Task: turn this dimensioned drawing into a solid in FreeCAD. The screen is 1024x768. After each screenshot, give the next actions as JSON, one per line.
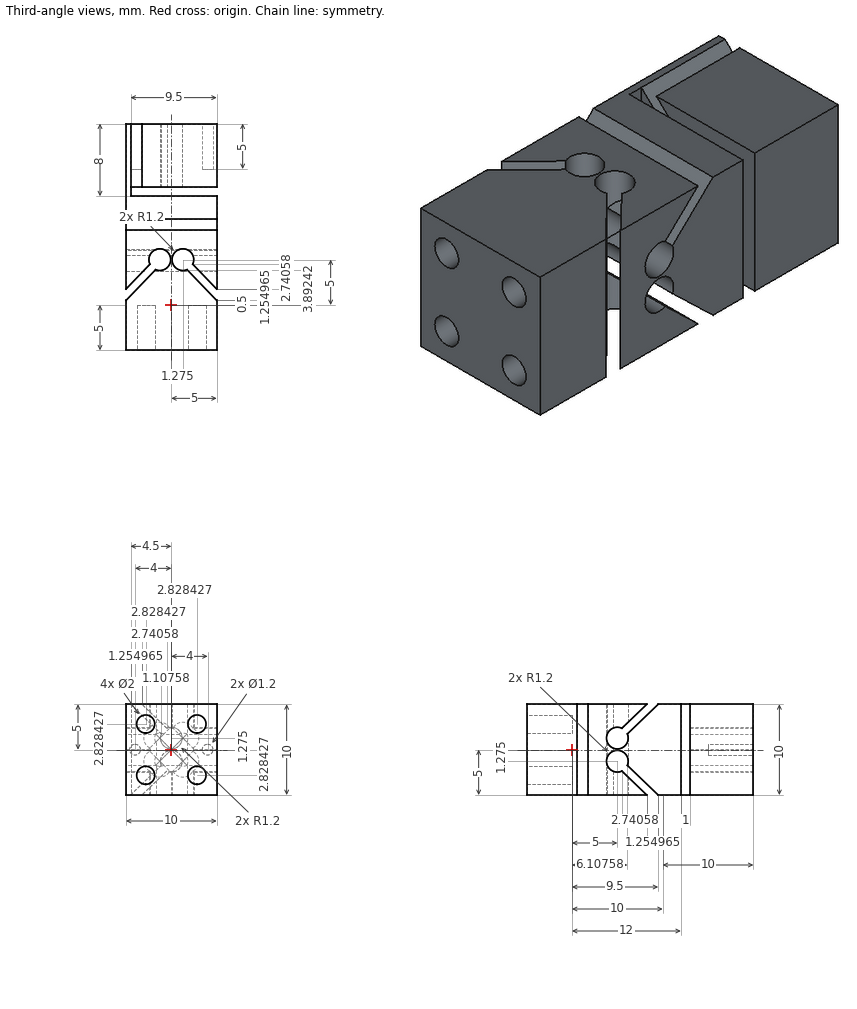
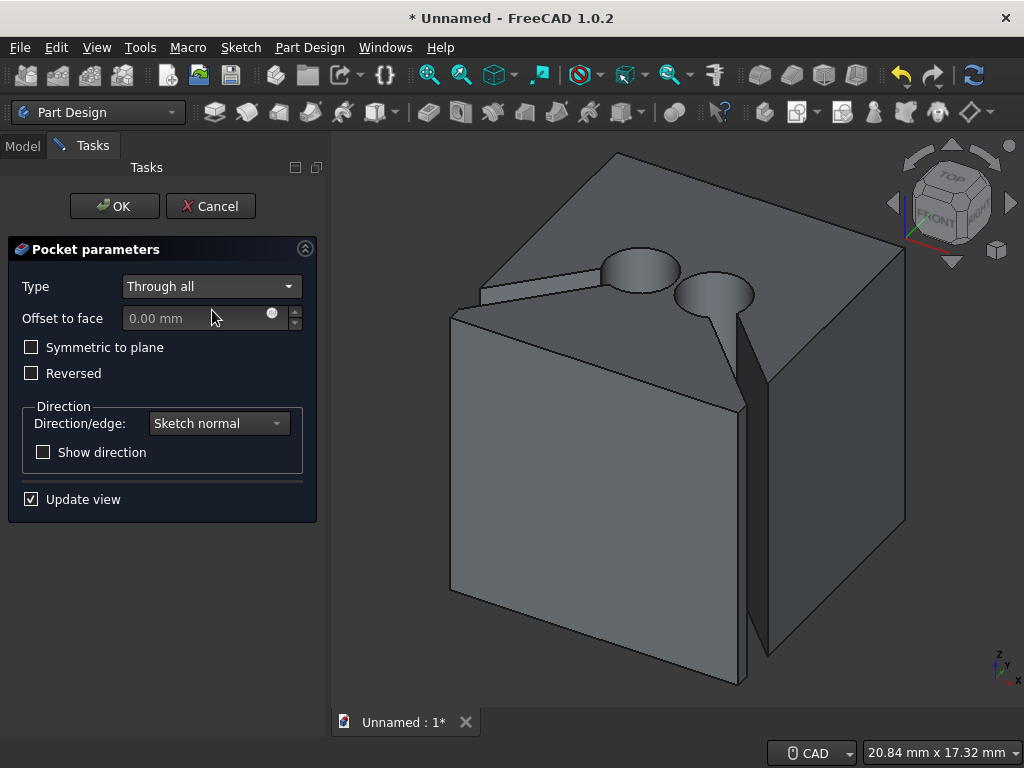
{"action": "left_click", "coordinate": [115, 206]}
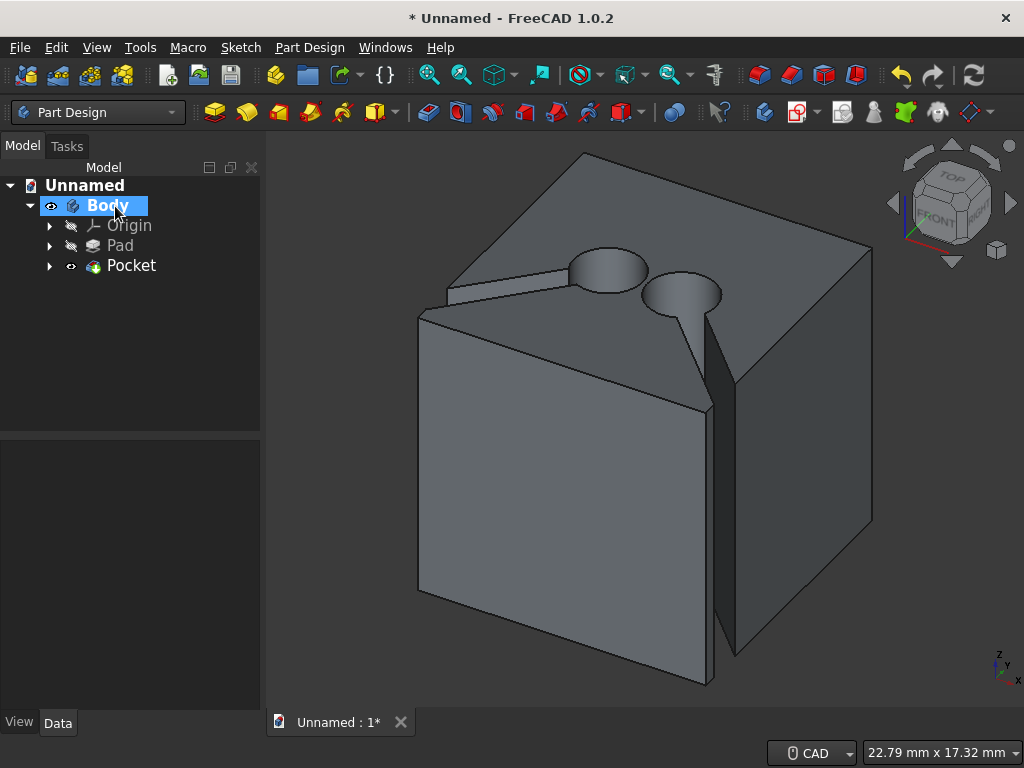
{"action": "left_click", "coordinate": [804, 451]}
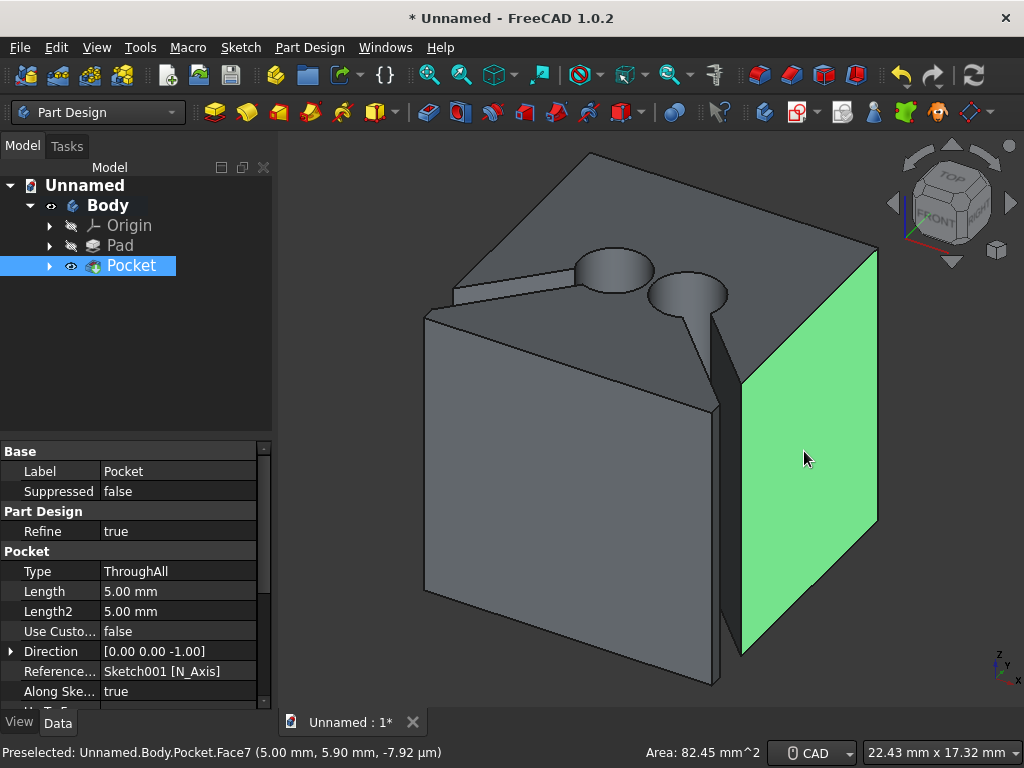
{"action": "left_click", "coordinate": [798, 112]}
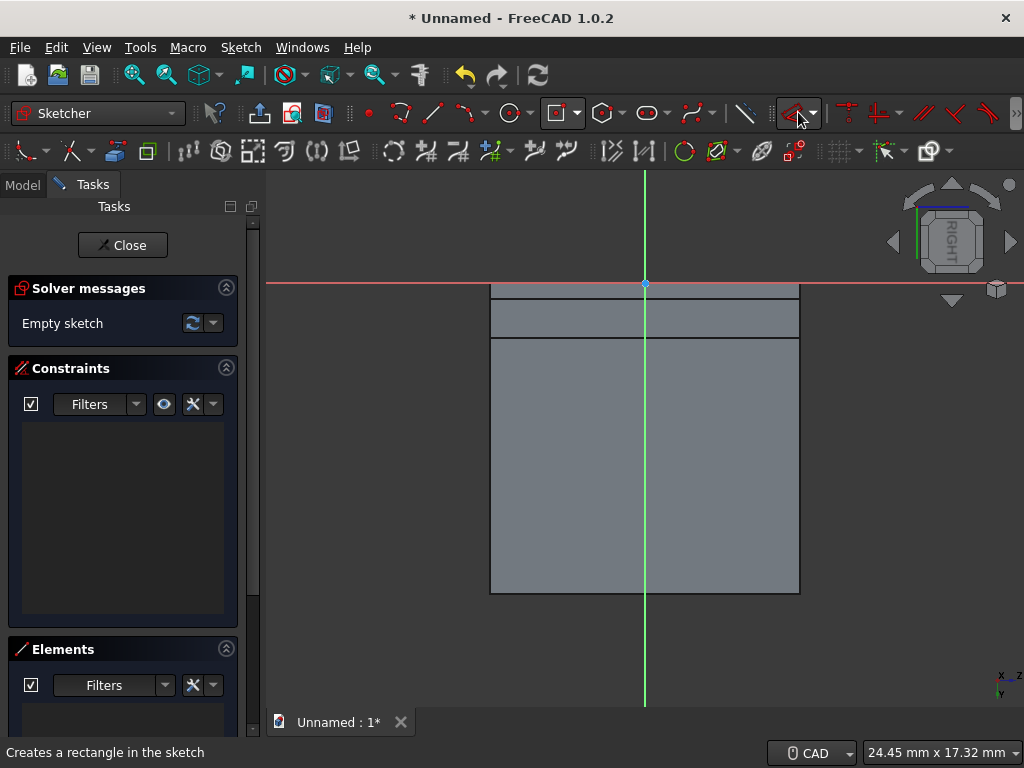
{"action": "left_click", "coordinate": [402, 114]}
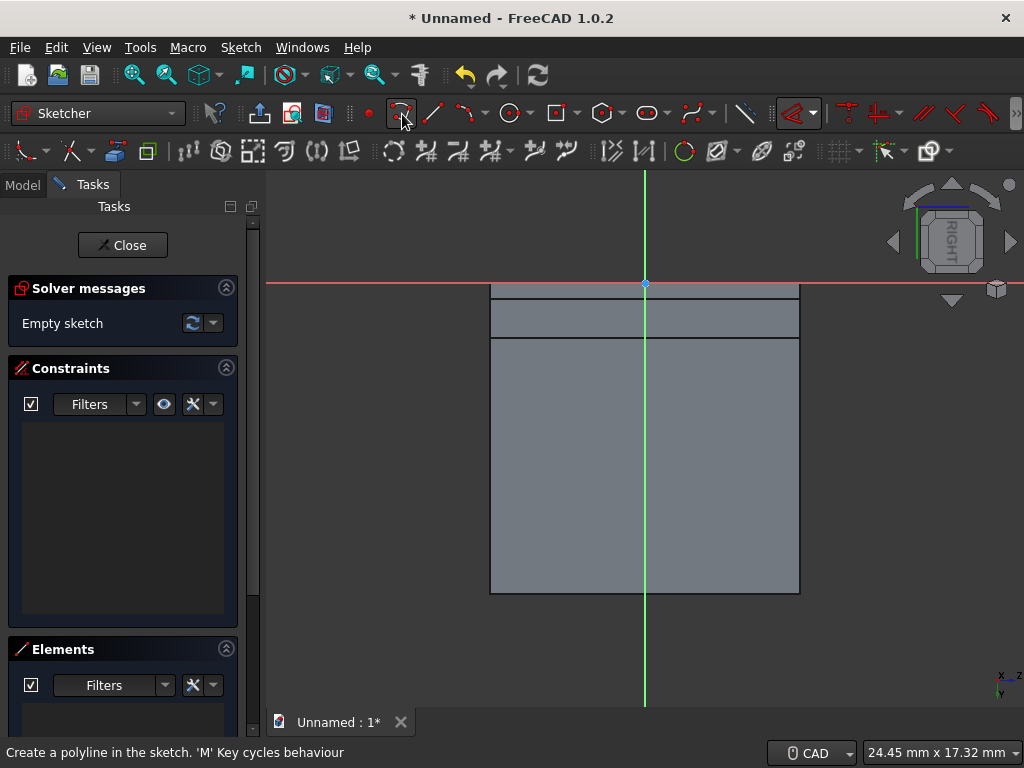
{"action": "left_click", "coordinate": [572, 454]}
{"action": "left_click", "coordinate": [490, 539]}
{"action": "left_click", "coordinate": [490, 578]}
{"action": "left_click", "coordinate": [591, 473]}
{"action": "right_click", "coordinate": [591, 473]}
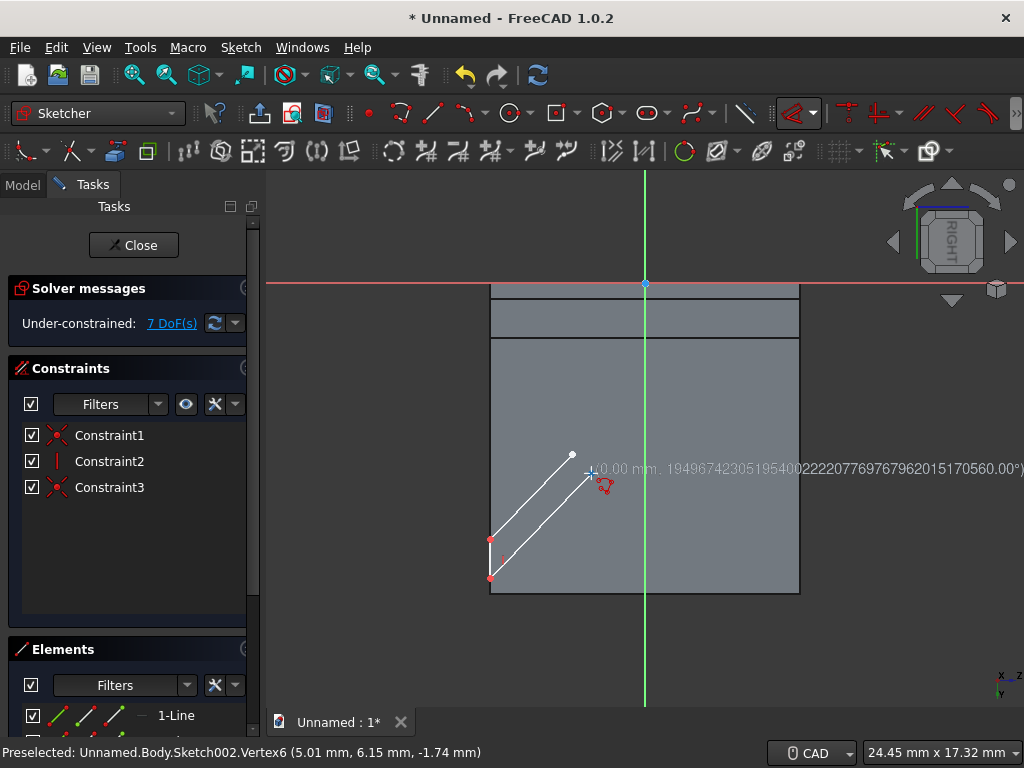
{"action": "left_click", "coordinate": [466, 114]}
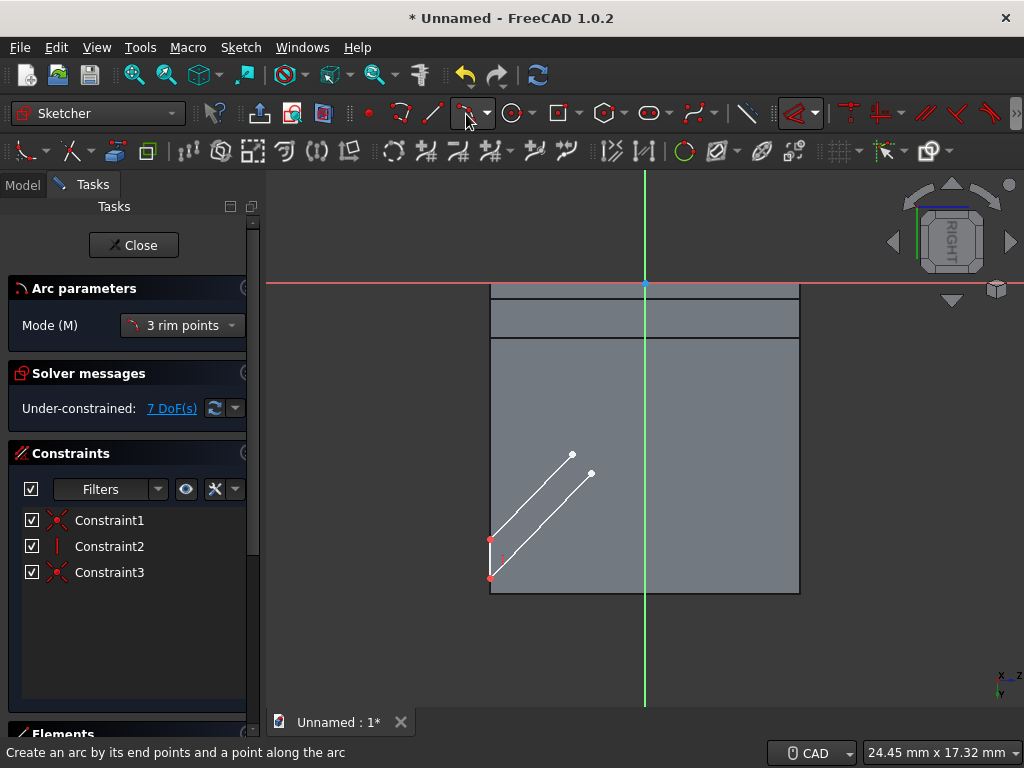
{"action": "left_click", "coordinate": [591, 474]}
{"action": "left_click", "coordinate": [572, 455]}
{"action": "left_click", "coordinate": [613, 402]}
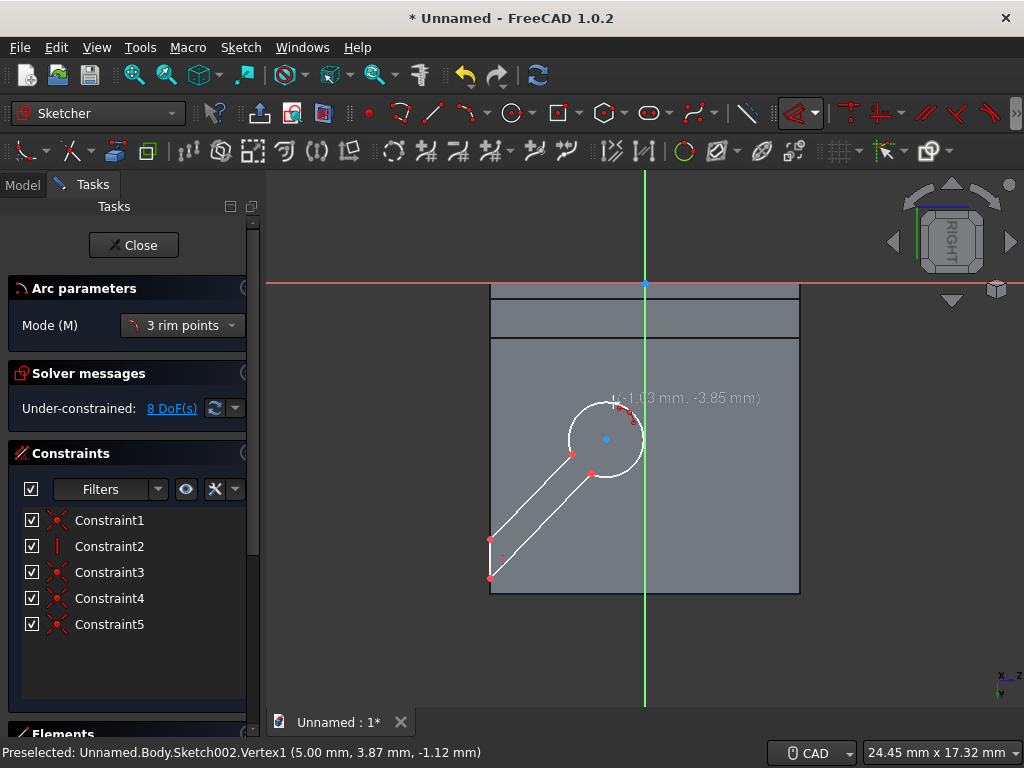
{"action": "left_click", "coordinate": [402, 114]}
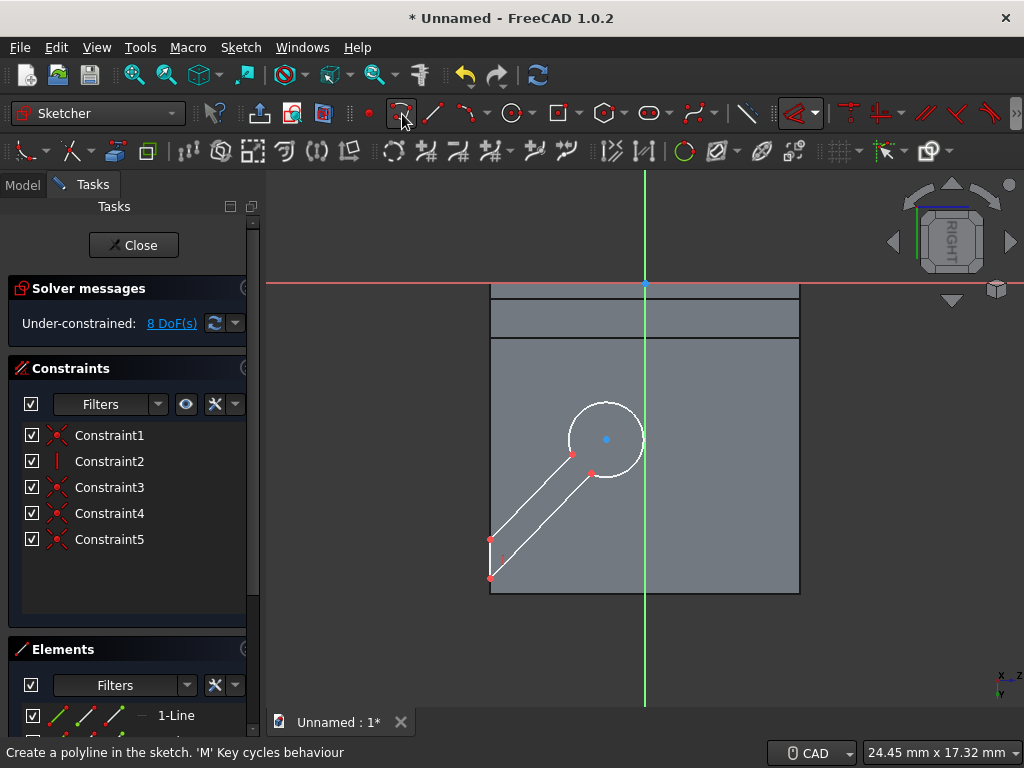
{"action": "left_click", "coordinate": [699, 473]}
{"action": "left_click", "coordinate": [800, 578]}
{"action": "left_click", "coordinate": [800, 539]}
{"action": "left_click", "coordinate": [718, 454]}
{"action": "right_click", "coordinate": [718, 454]}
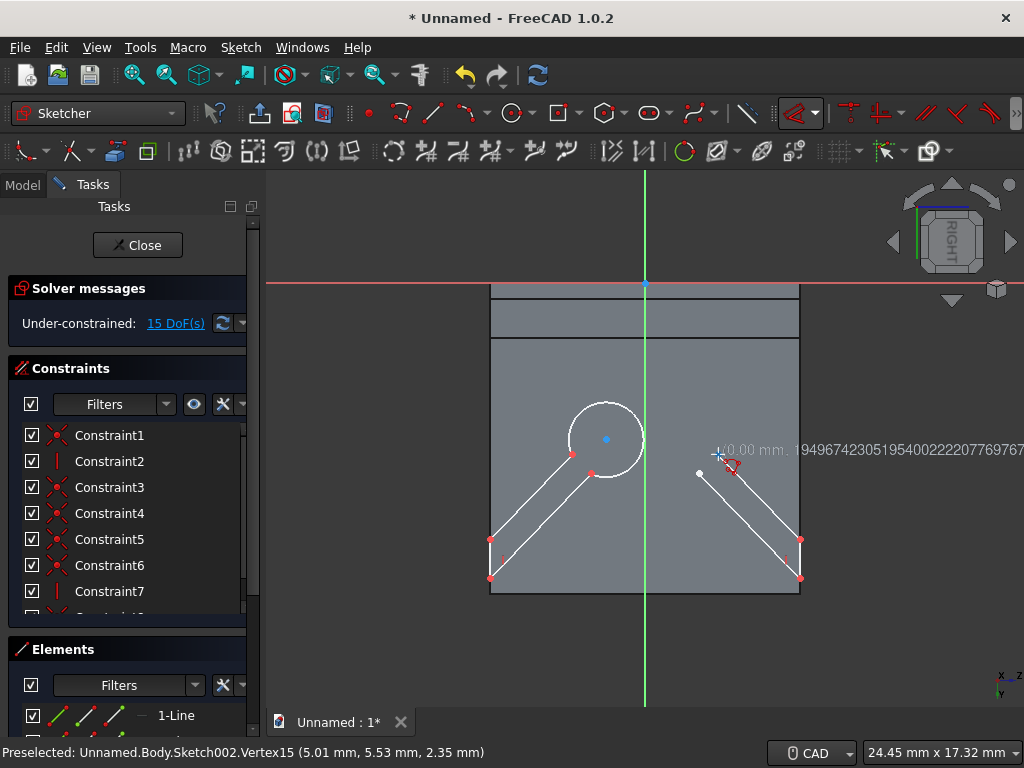
{"action": "left_click", "coordinate": [466, 114]}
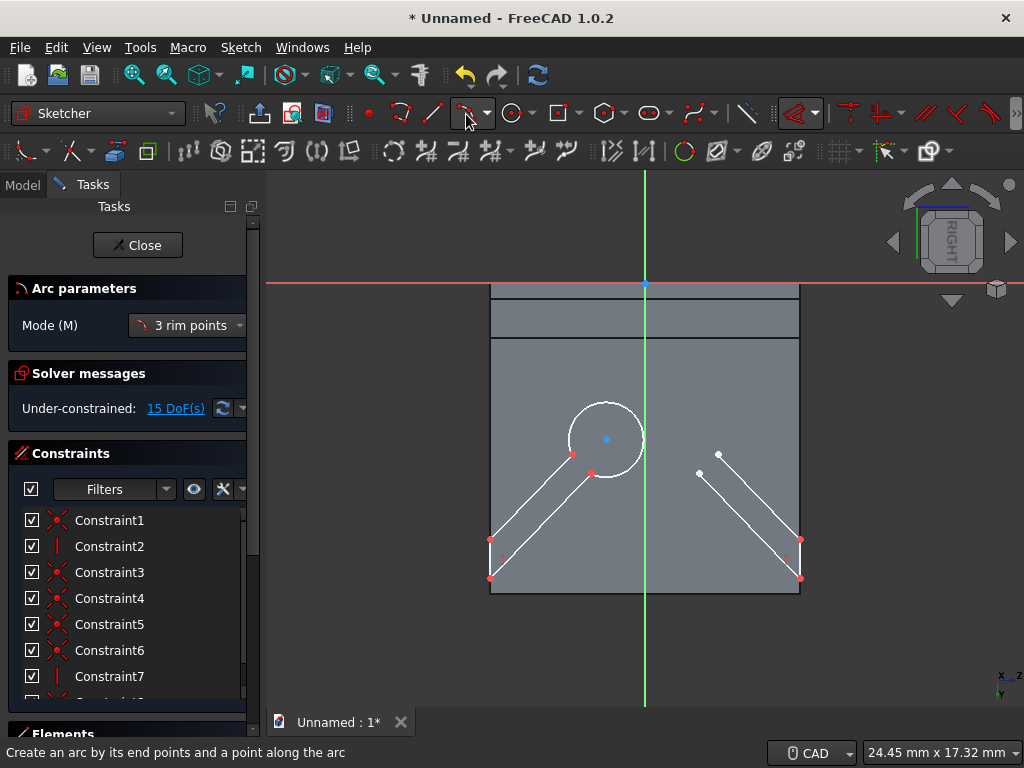
{"action": "left_click", "coordinate": [718, 455]}
{"action": "left_click", "coordinate": [699, 474]}
{"action": "left_click", "coordinate": [677, 402]}
{"action": "key", "text": "Escape"}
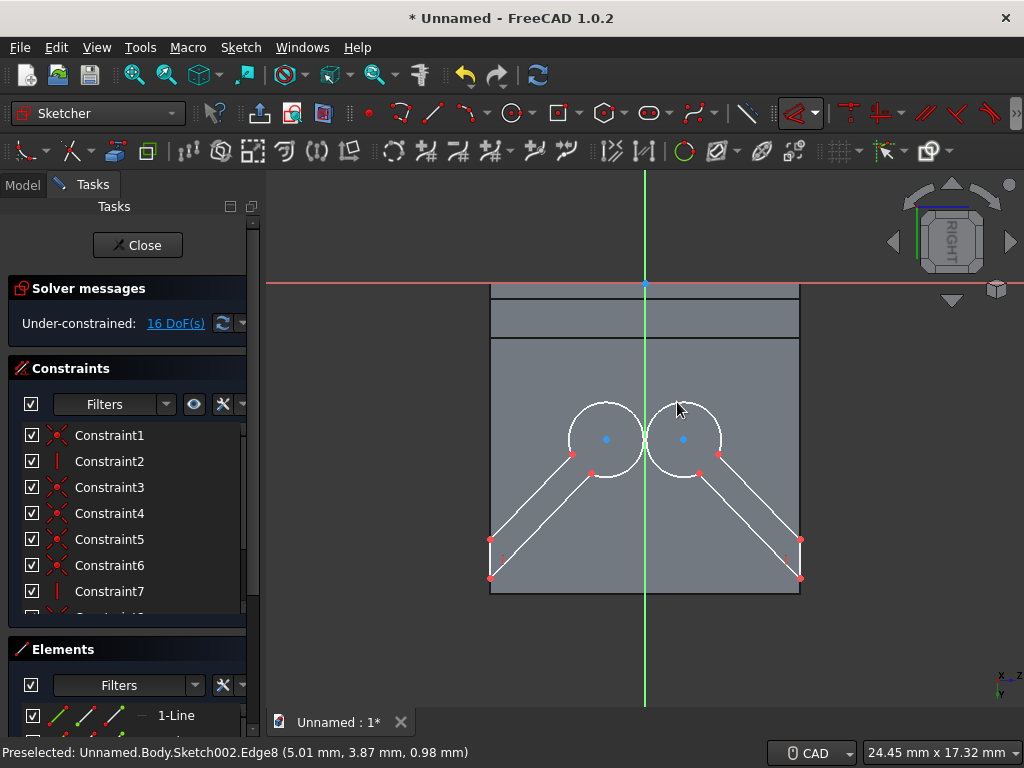
{"action": "left_click", "coordinate": [594, 404]}